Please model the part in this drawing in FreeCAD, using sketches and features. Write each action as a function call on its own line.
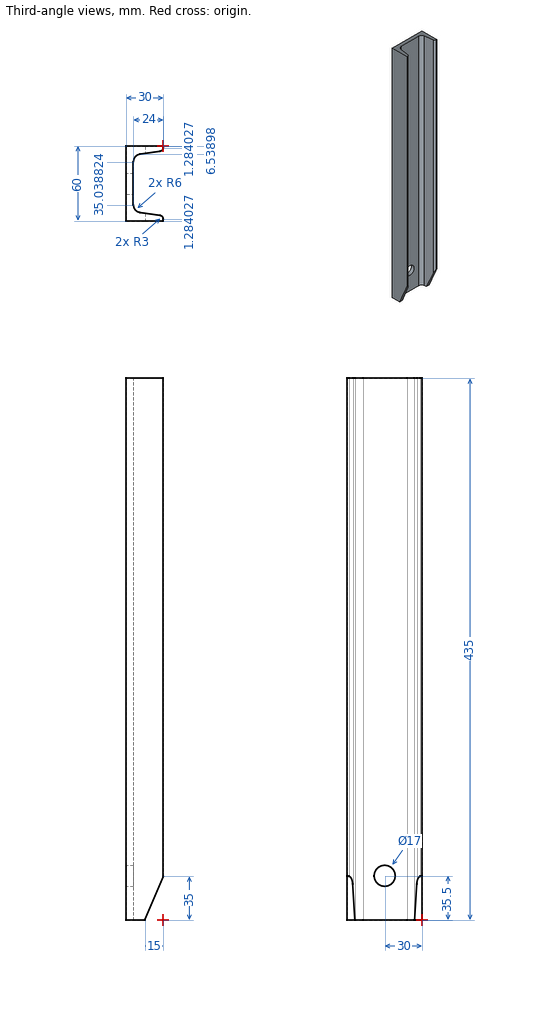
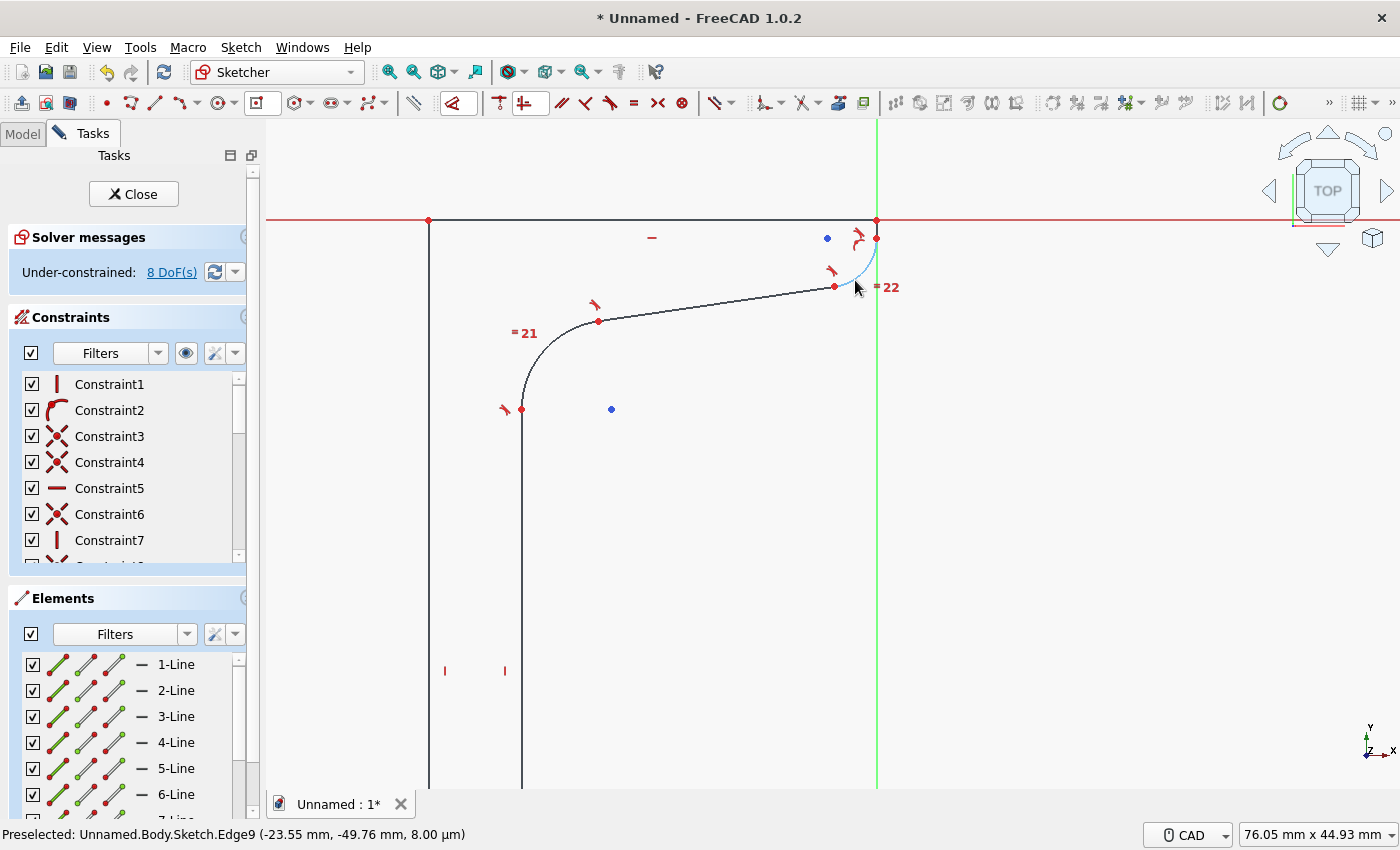
click(854, 280)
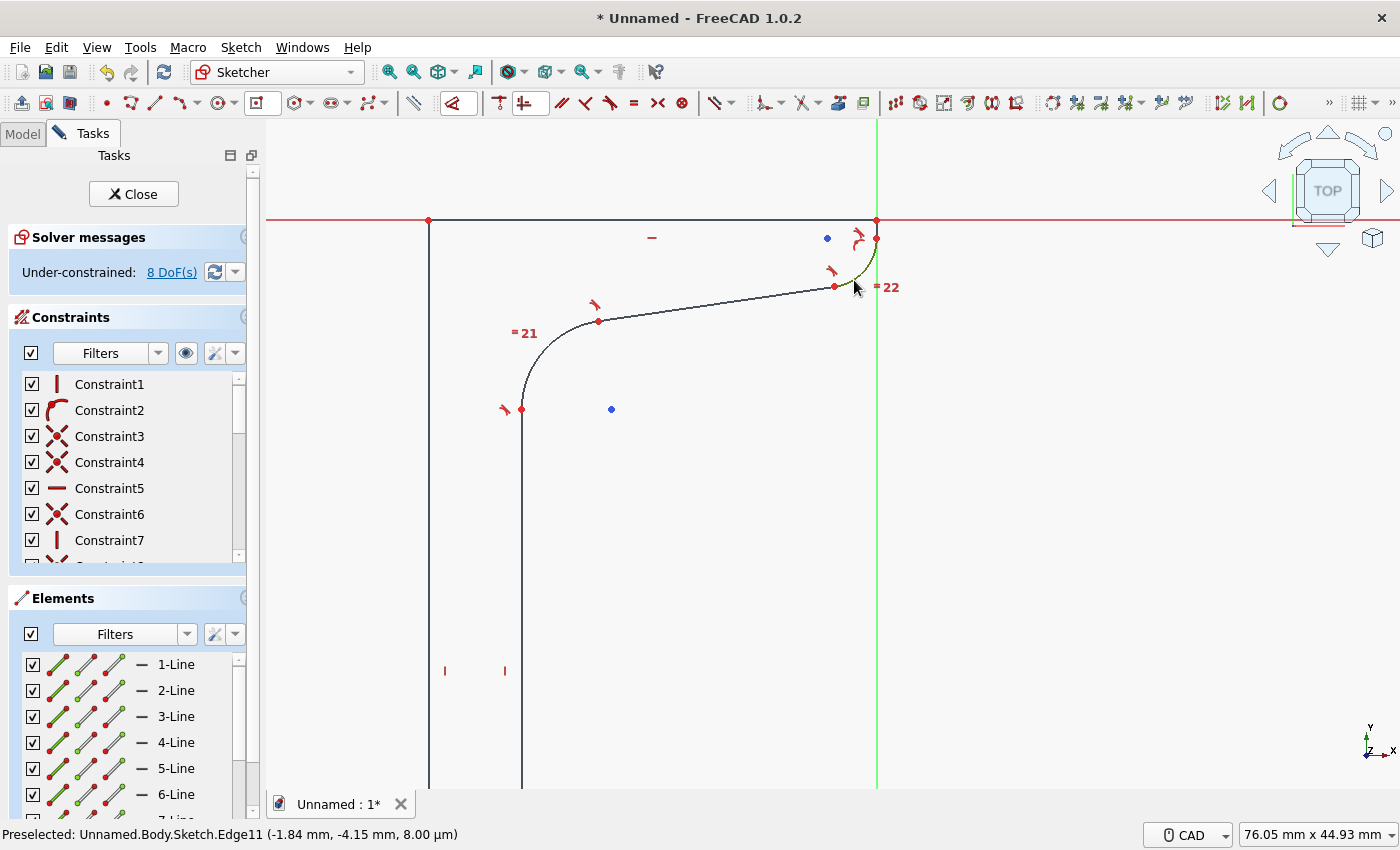
key(k)
key(r)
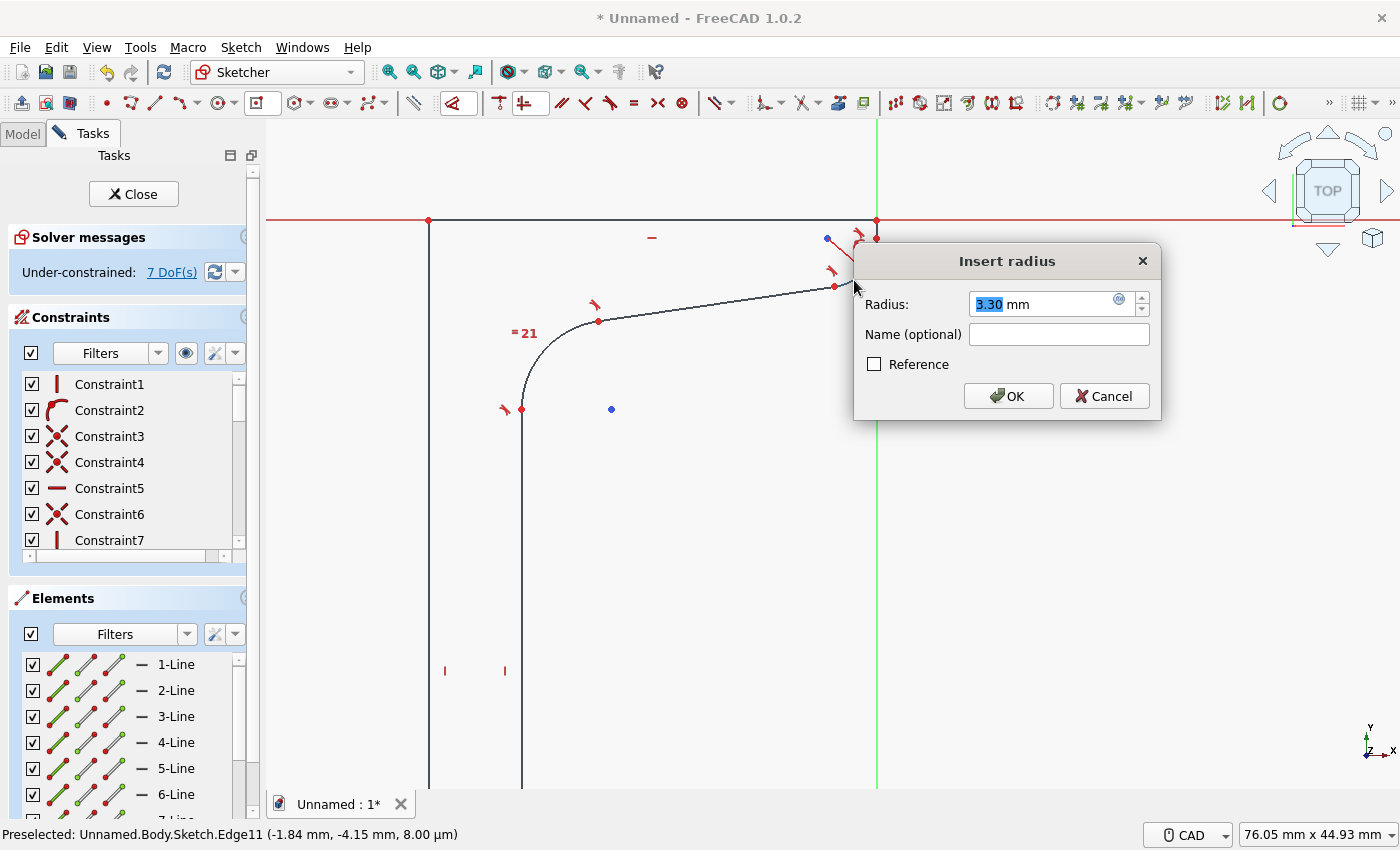
text(3)
key(Return)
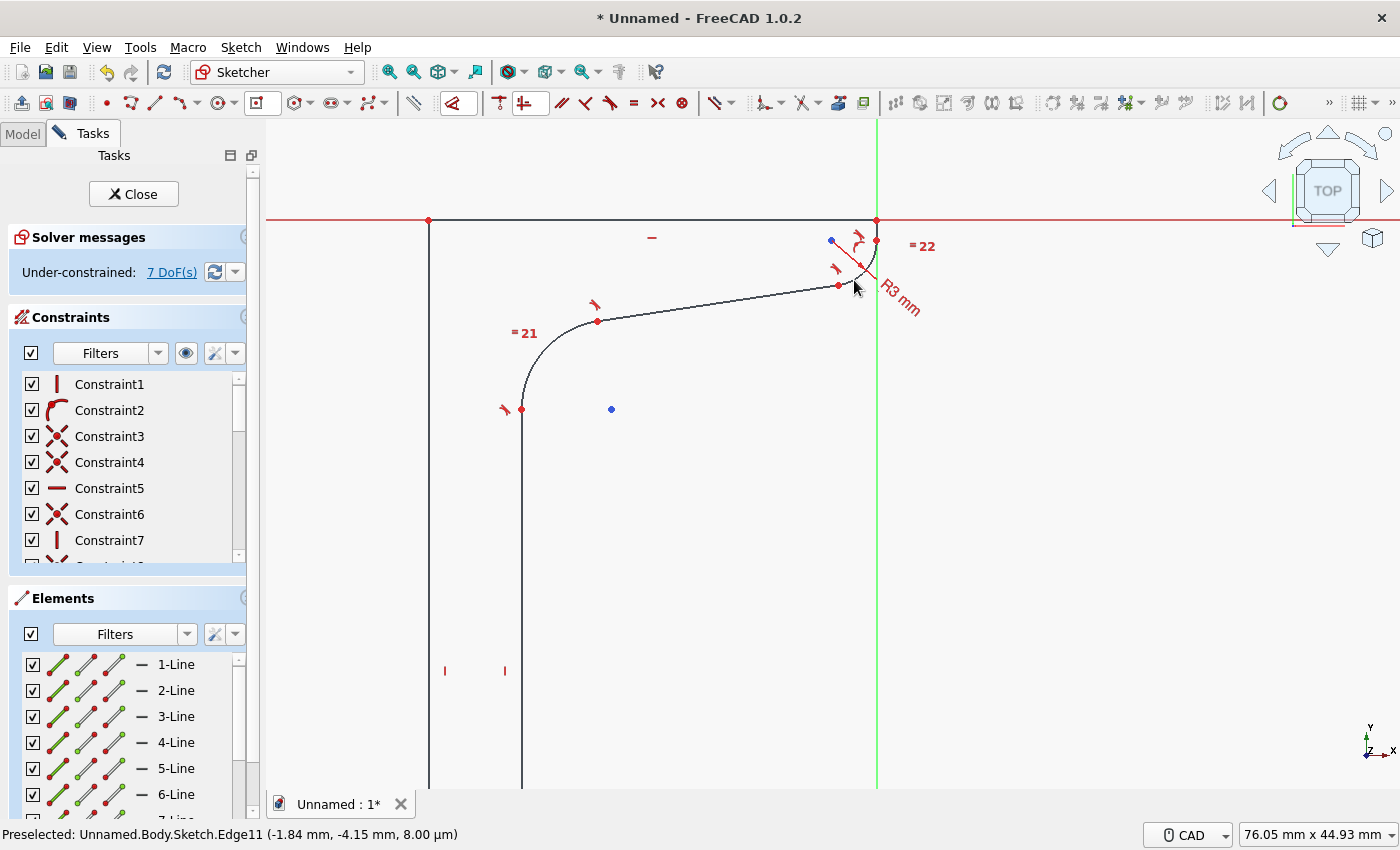
click(742, 220)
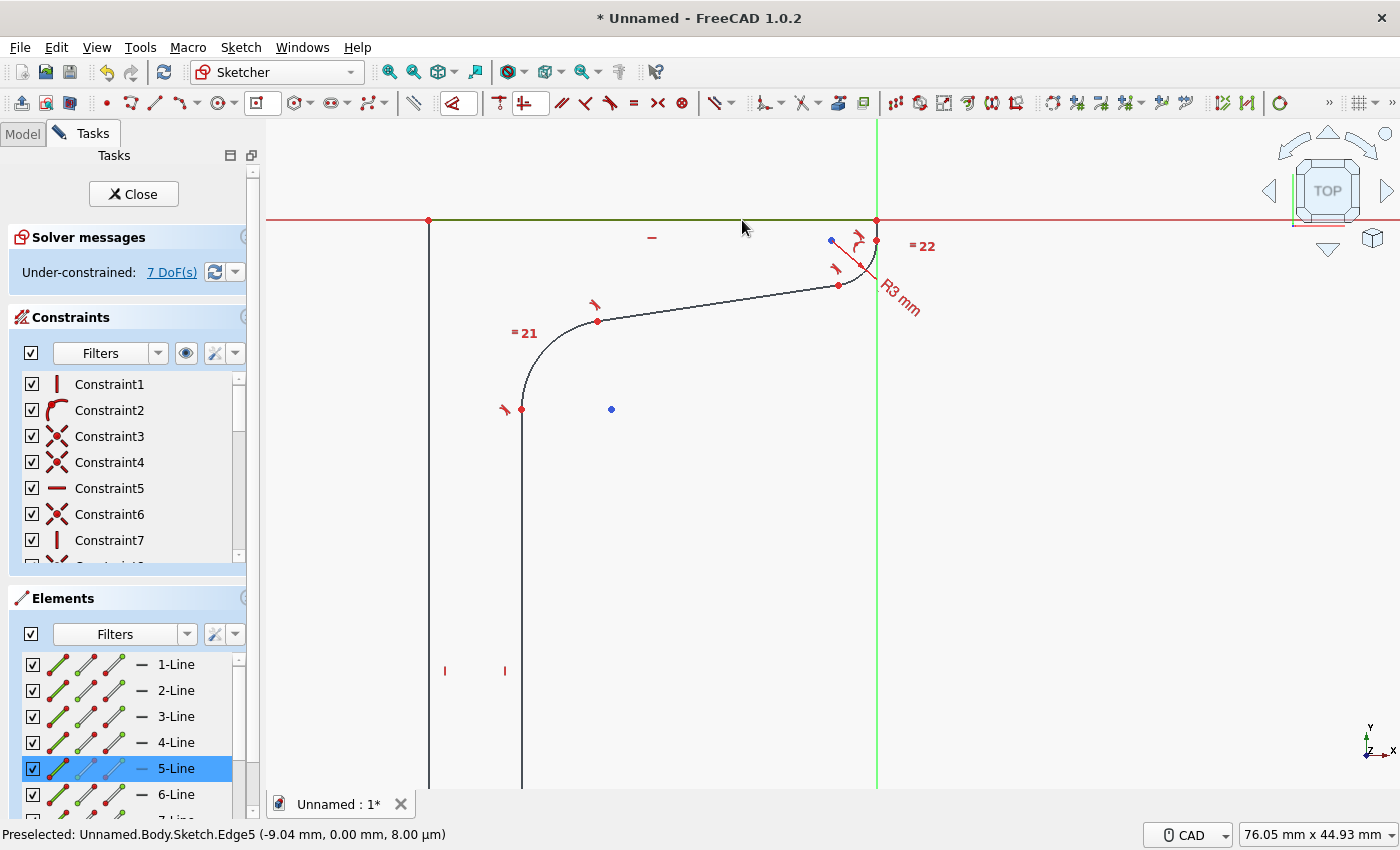
click(472, 104)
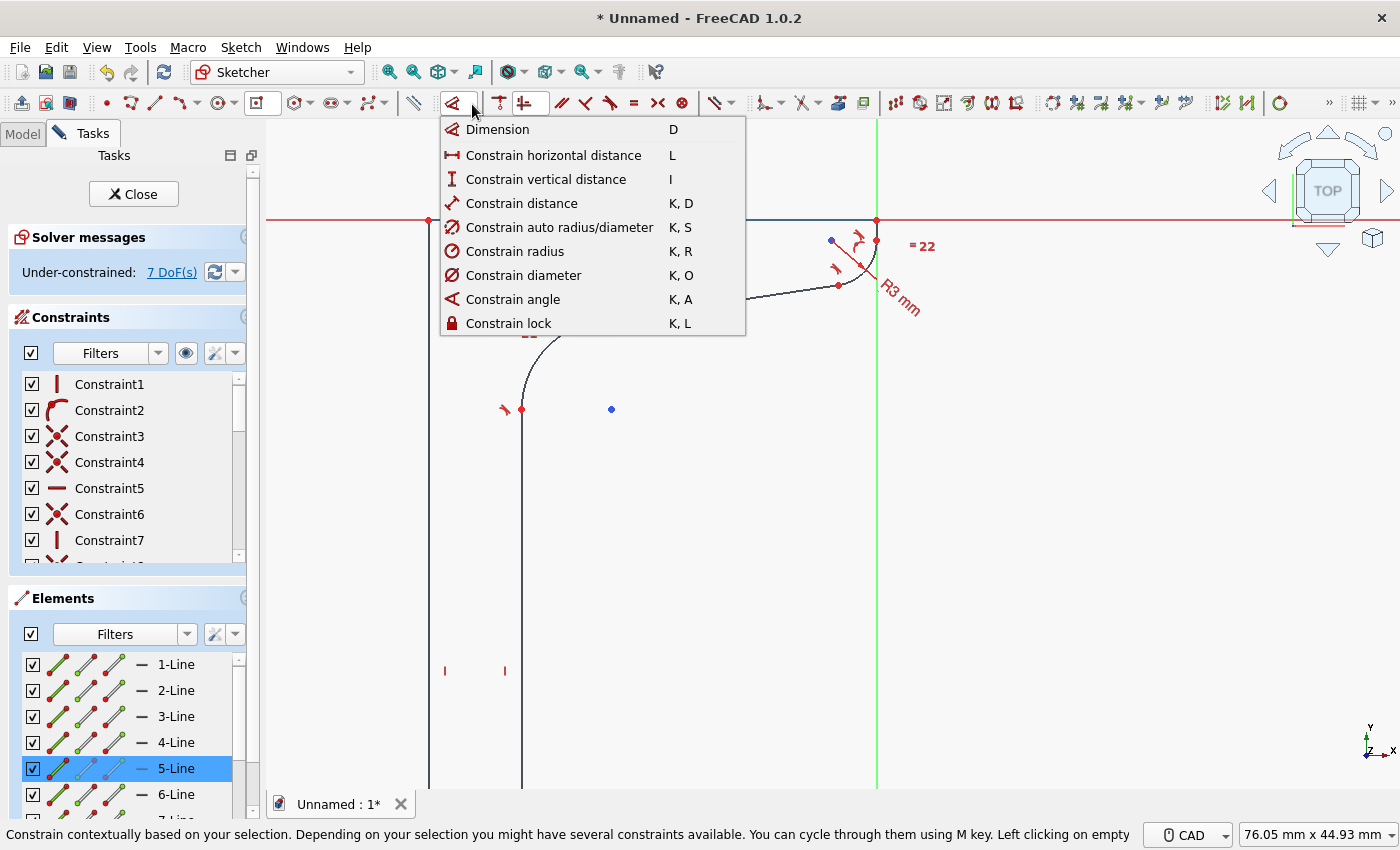
click(593, 155)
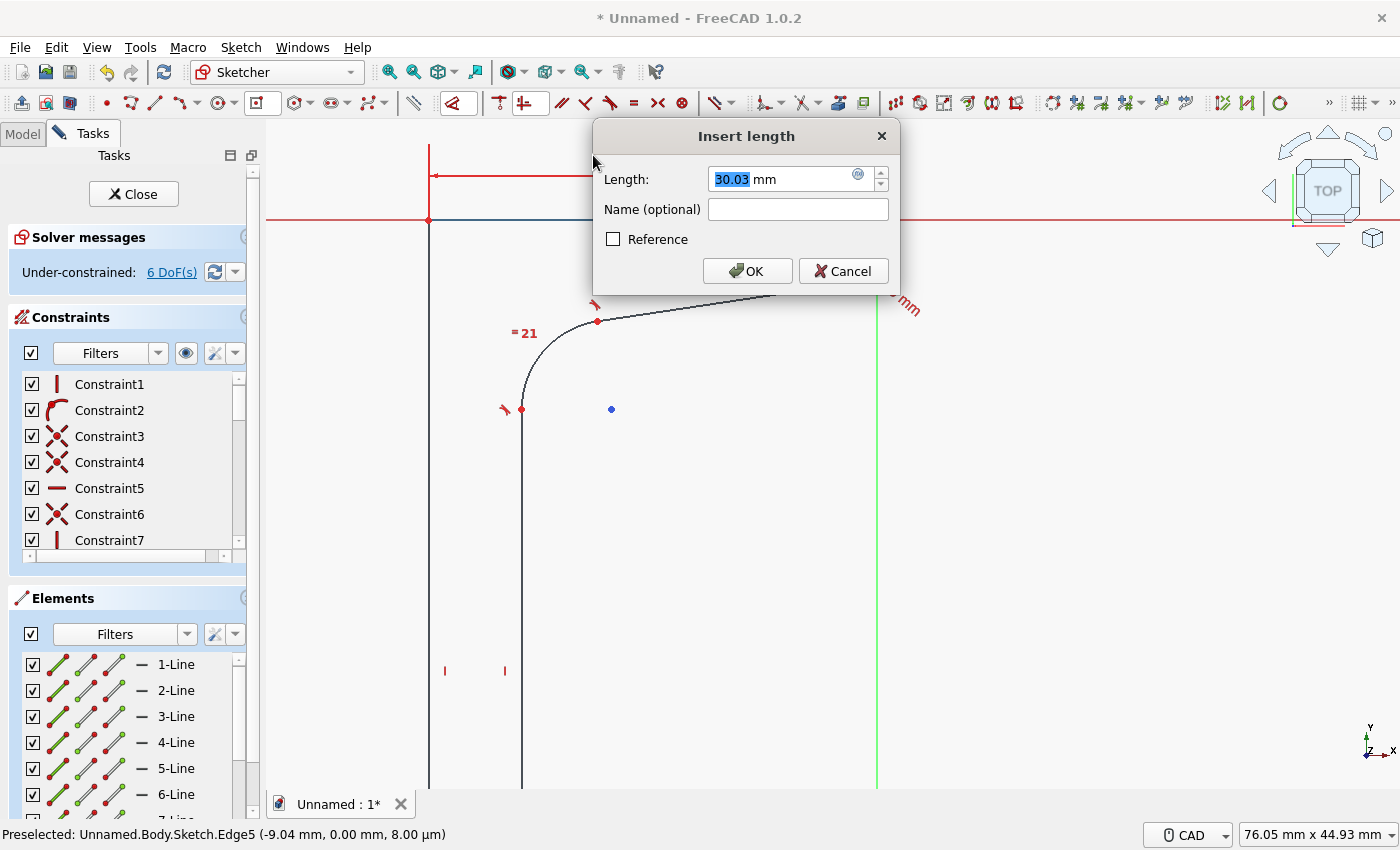
text(30)
key(Return)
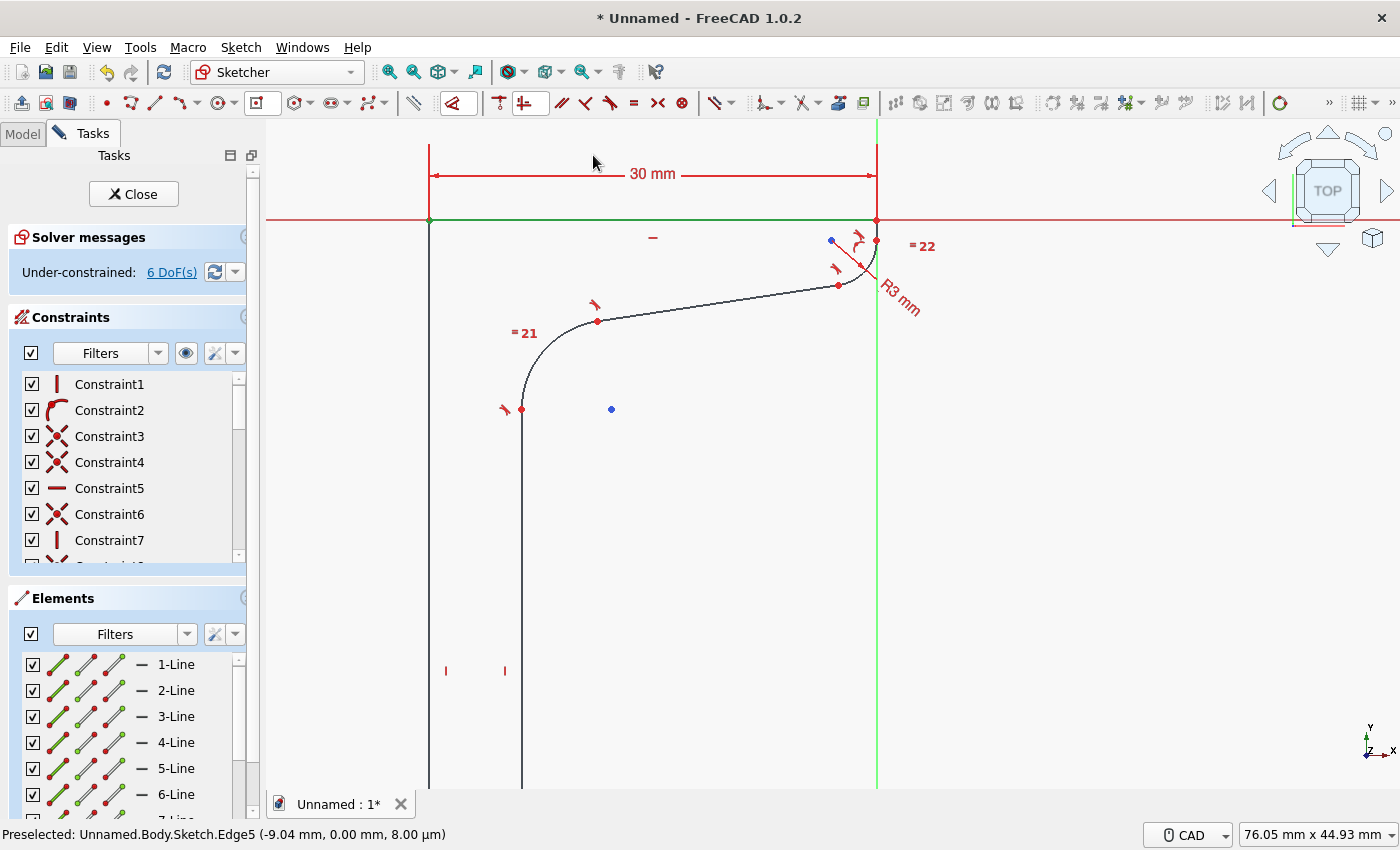
click(429, 490)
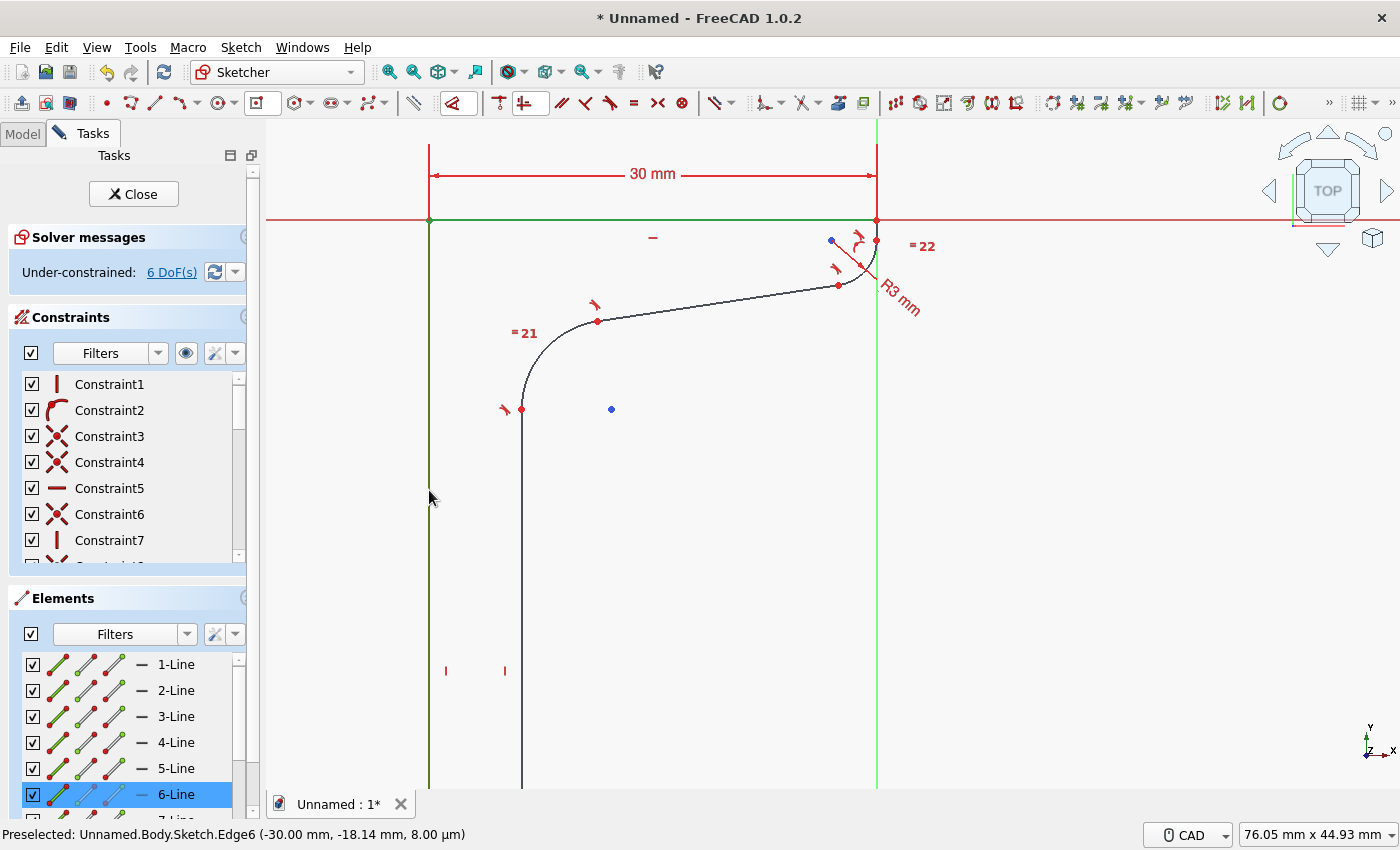
key(i)